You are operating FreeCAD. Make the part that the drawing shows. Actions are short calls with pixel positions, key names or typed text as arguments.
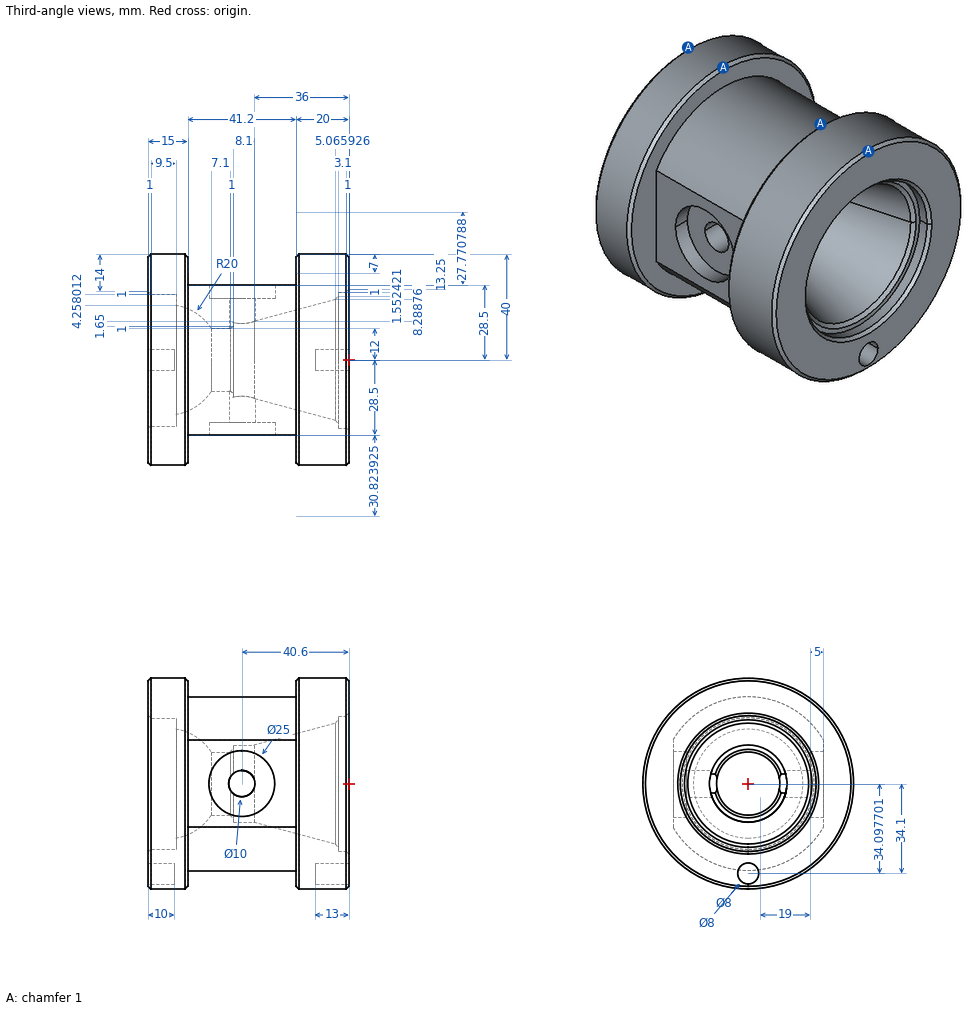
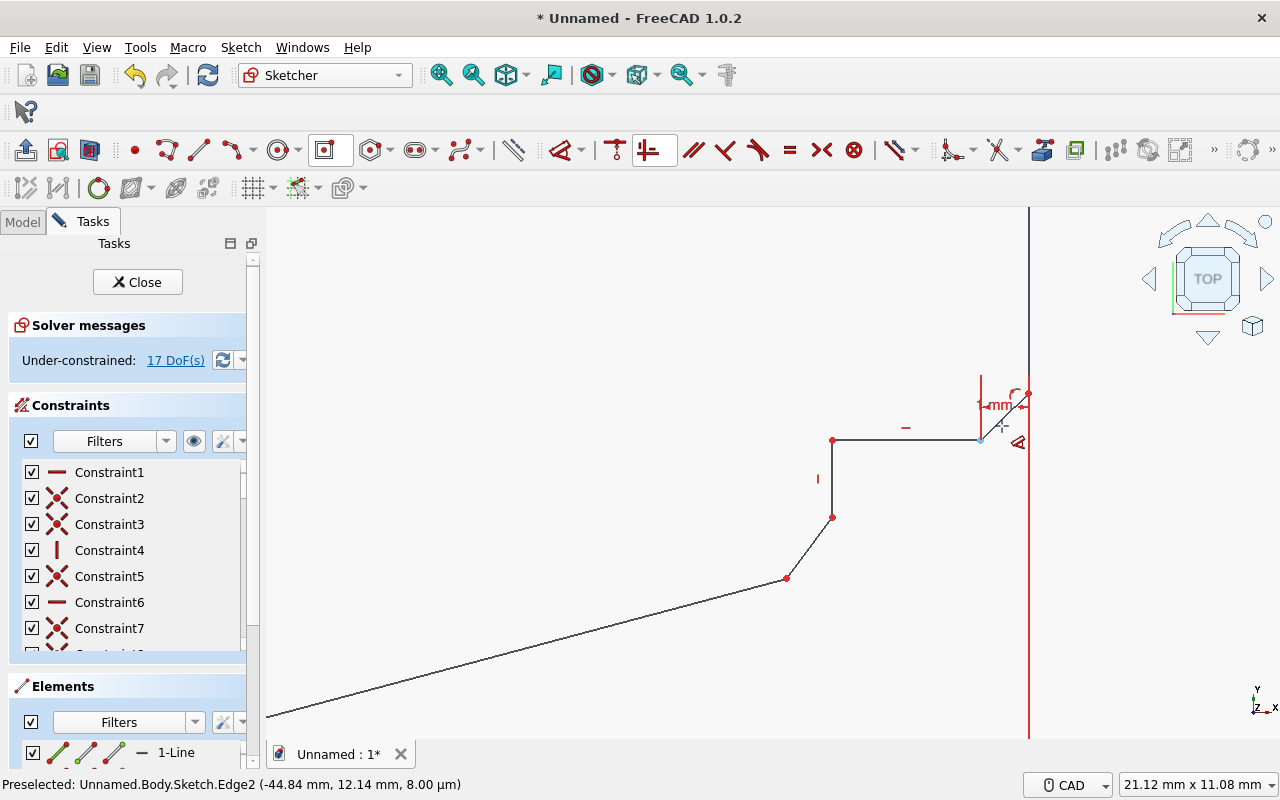
click(995, 426)
click(1063, 428)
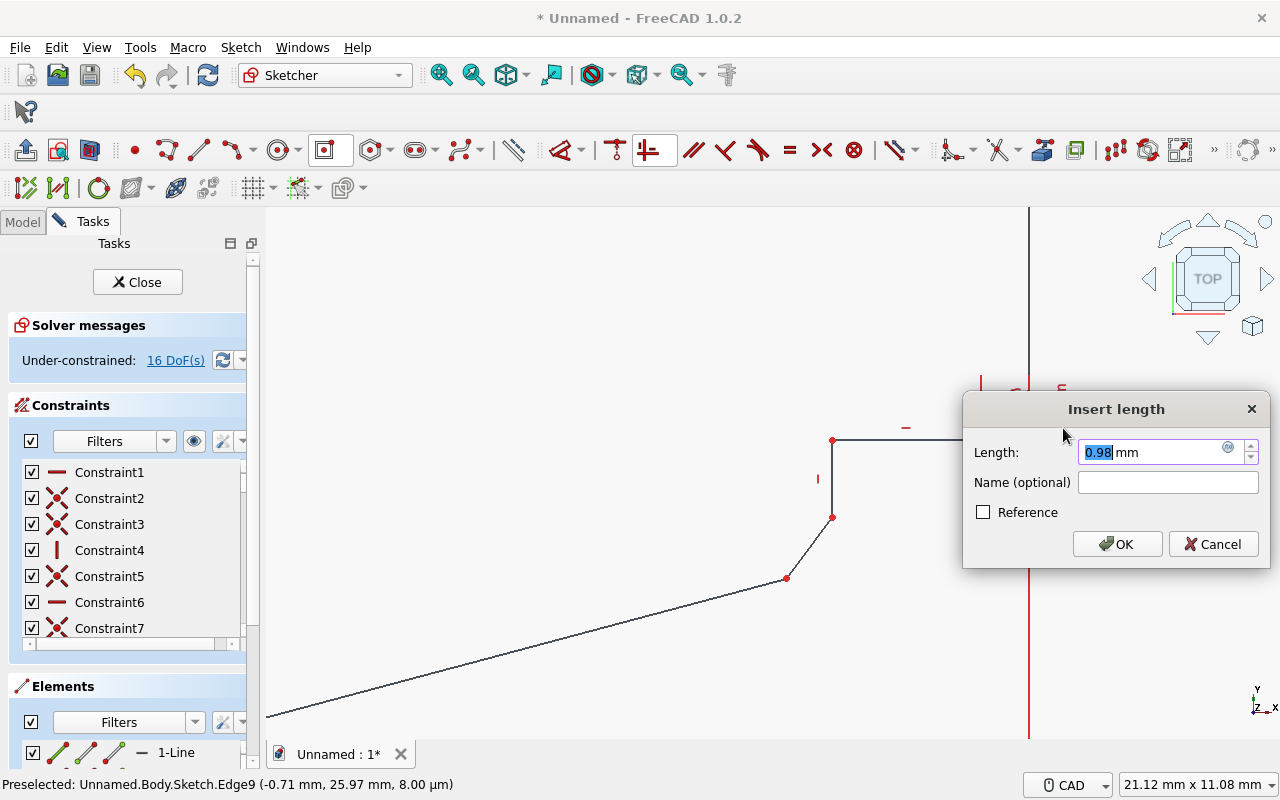
text(1)
key(Return)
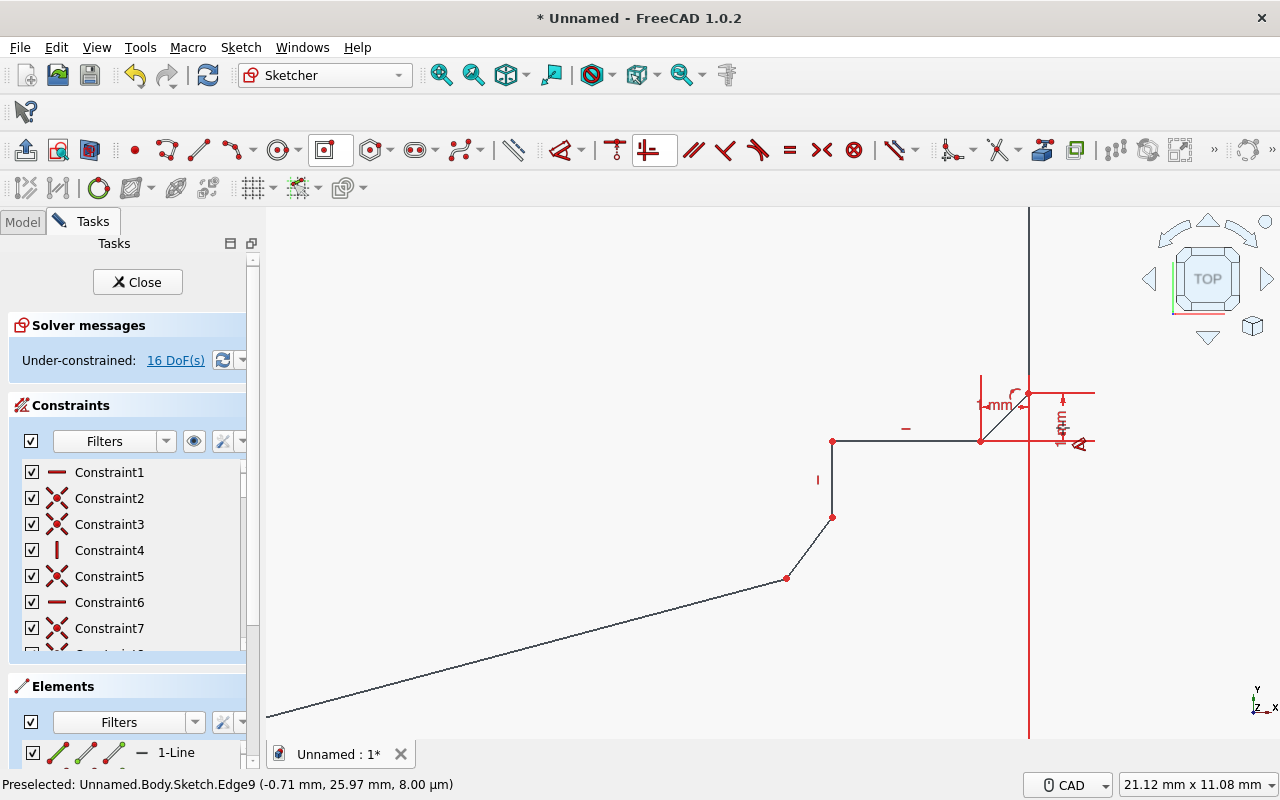
scroll(1003, 425, down, 9)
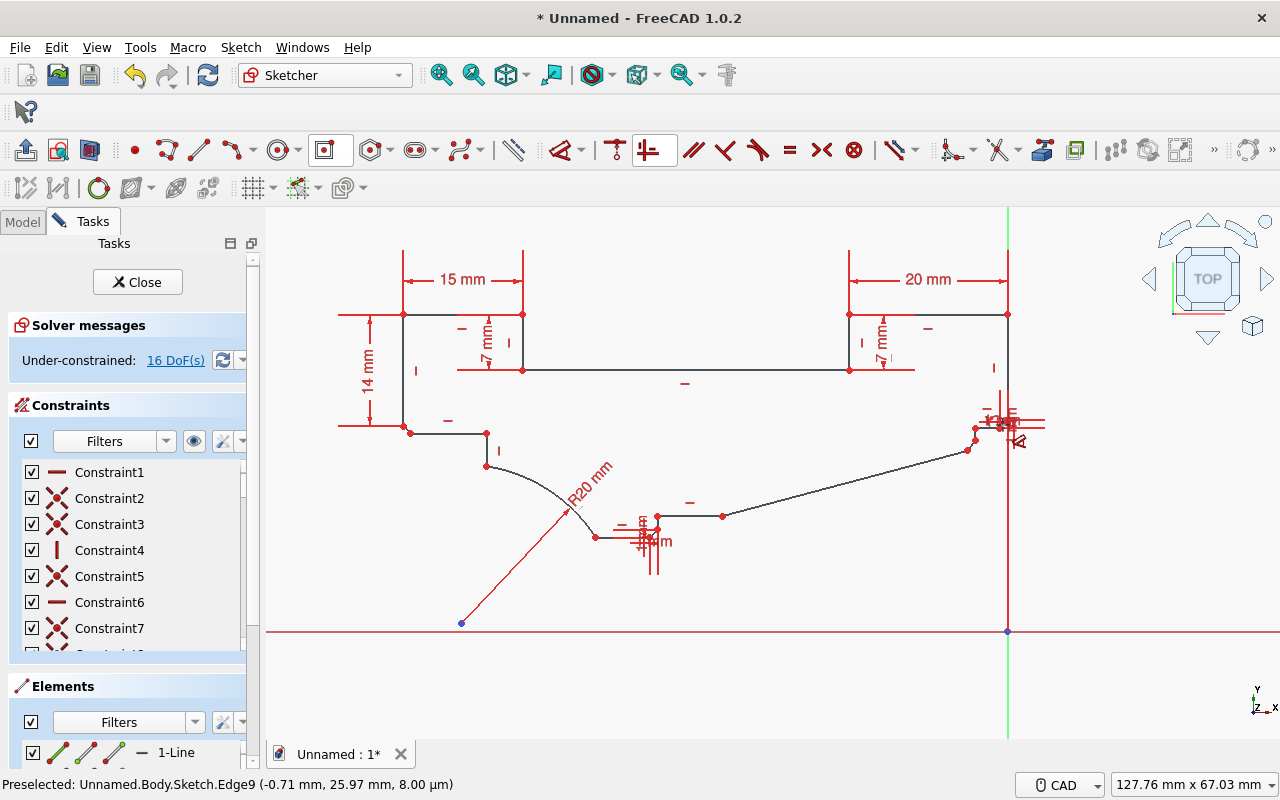
scroll(406, 428, up, 9)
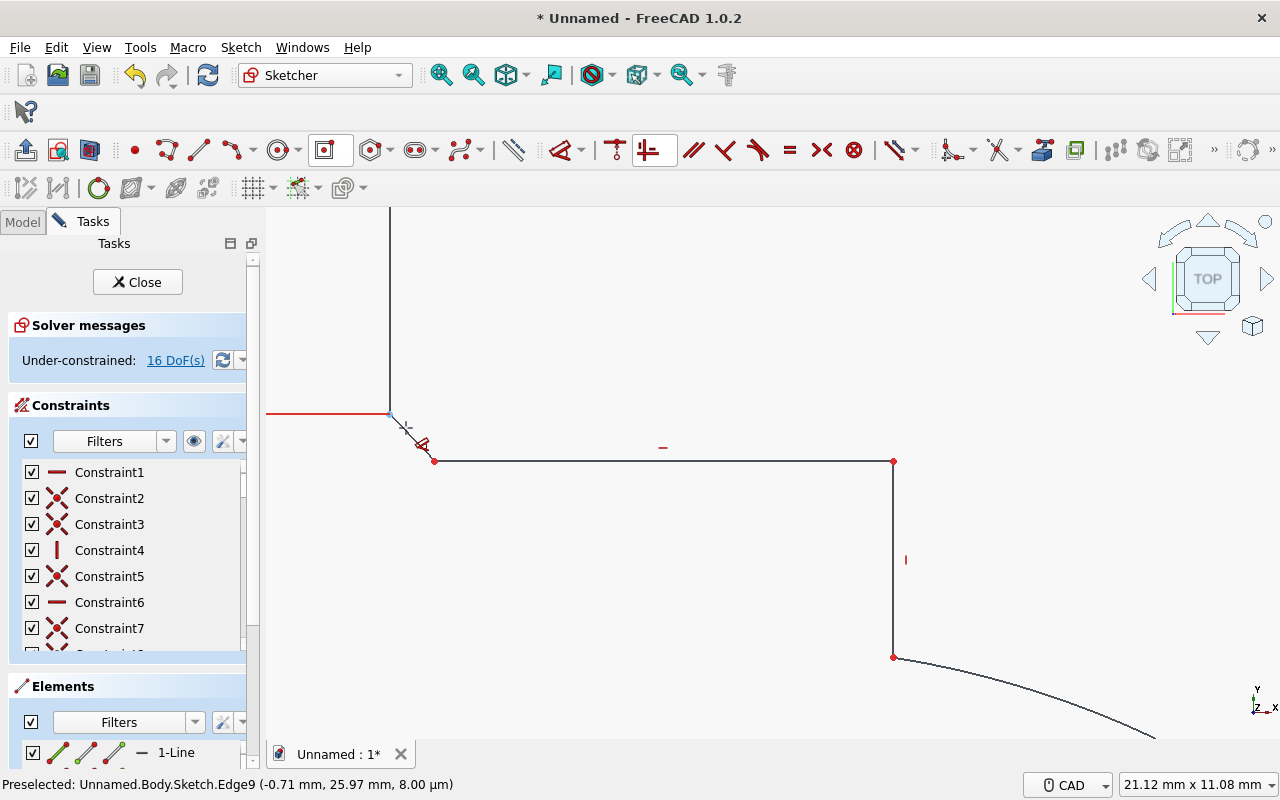
click(403, 428)
click(412, 380)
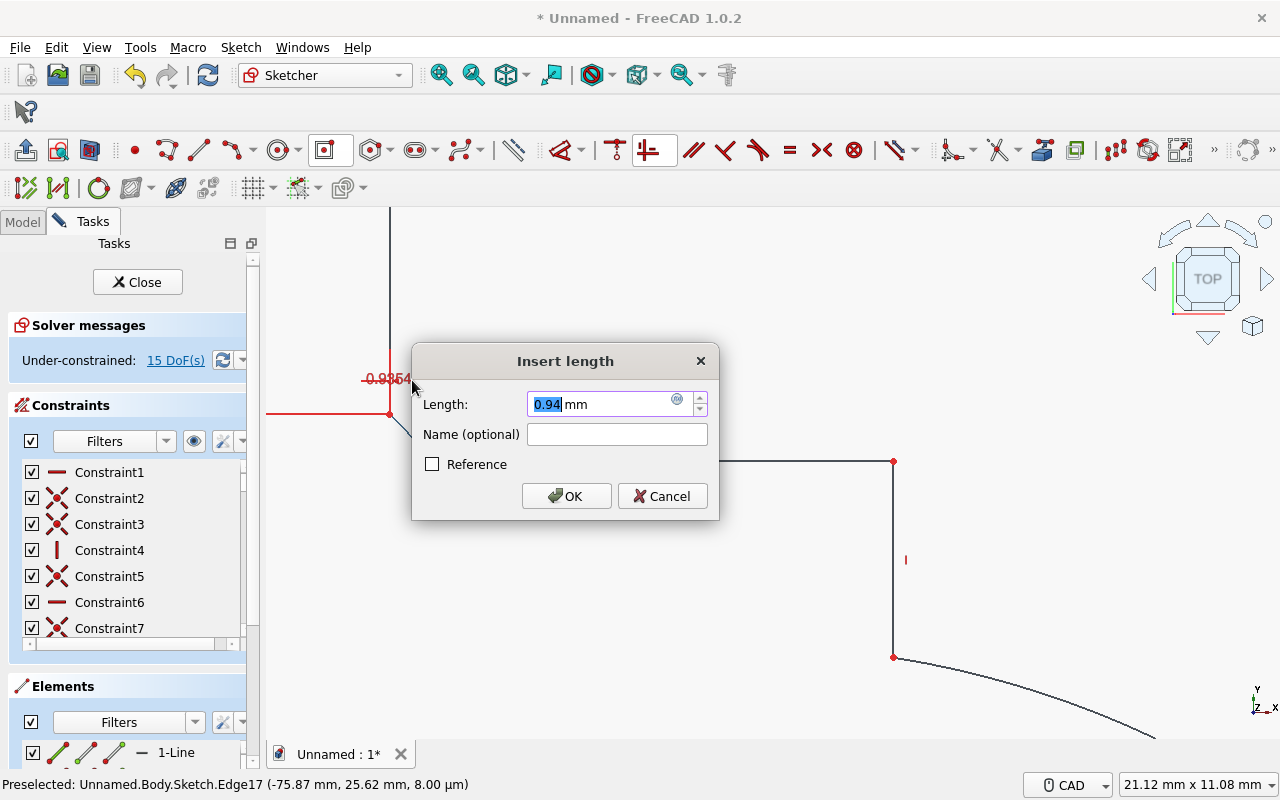
text(1)
key(Return)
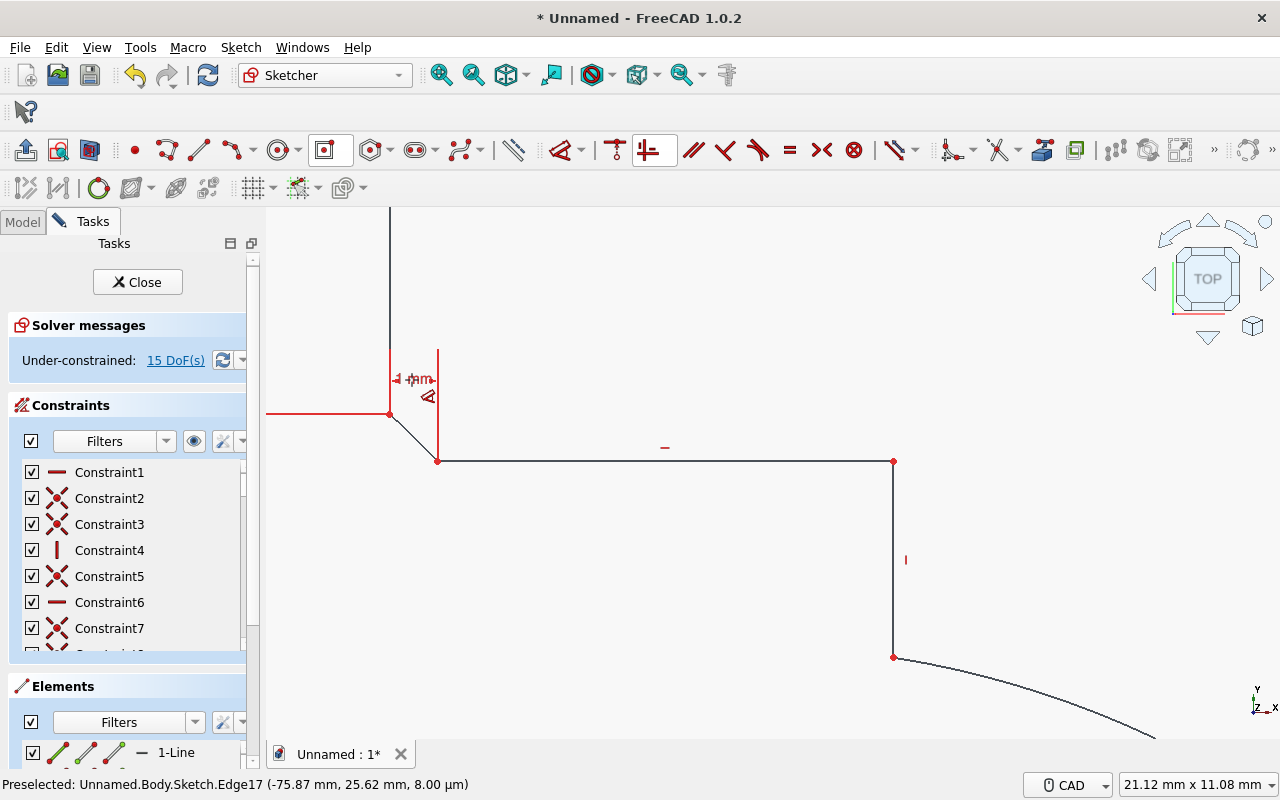
click(404, 428)
click(356, 438)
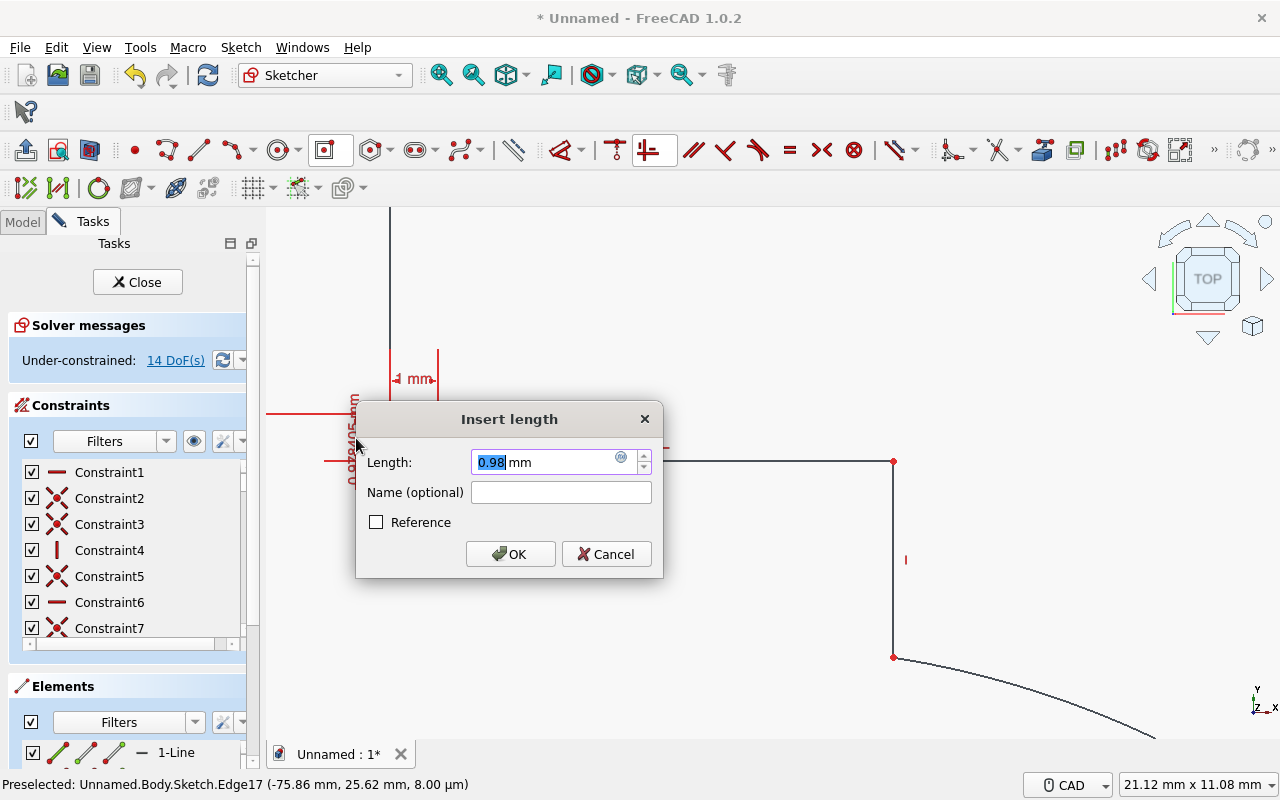
text(1)
key(Return)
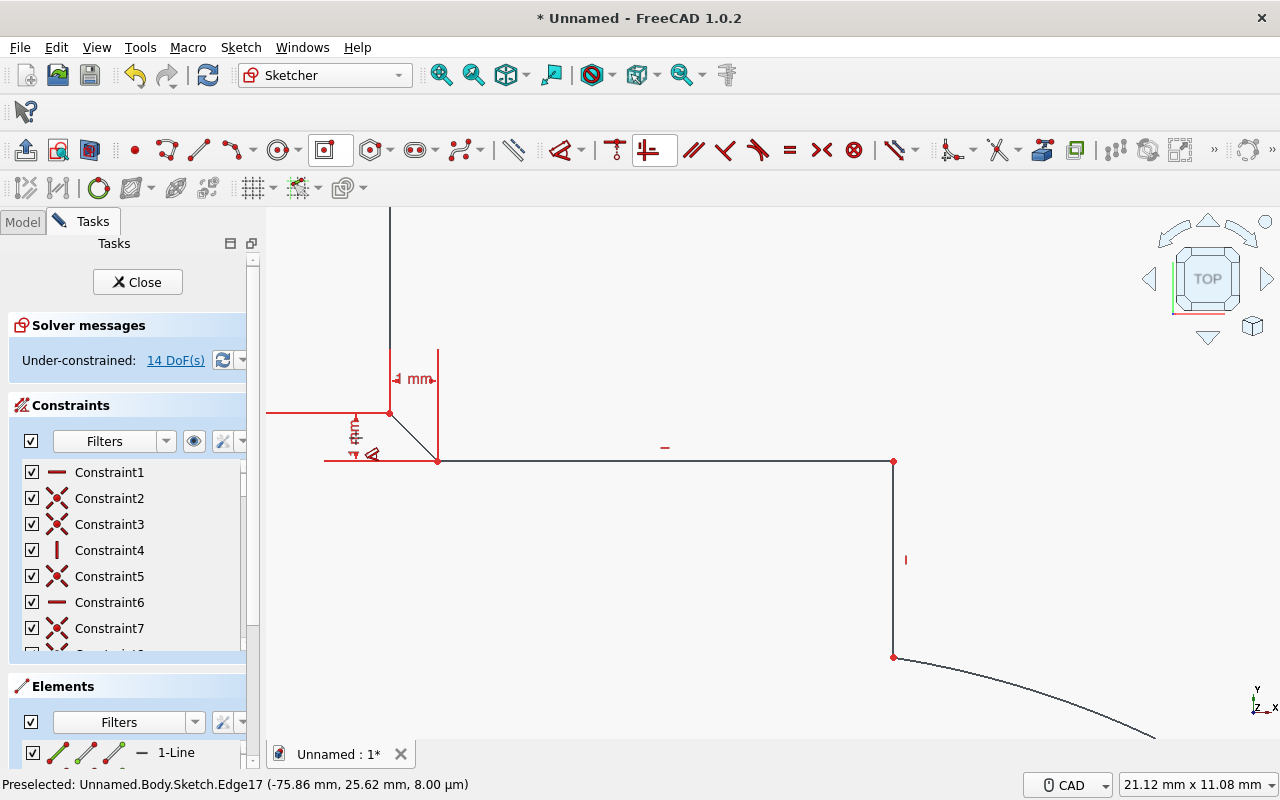
scroll(405, 428, down, 9)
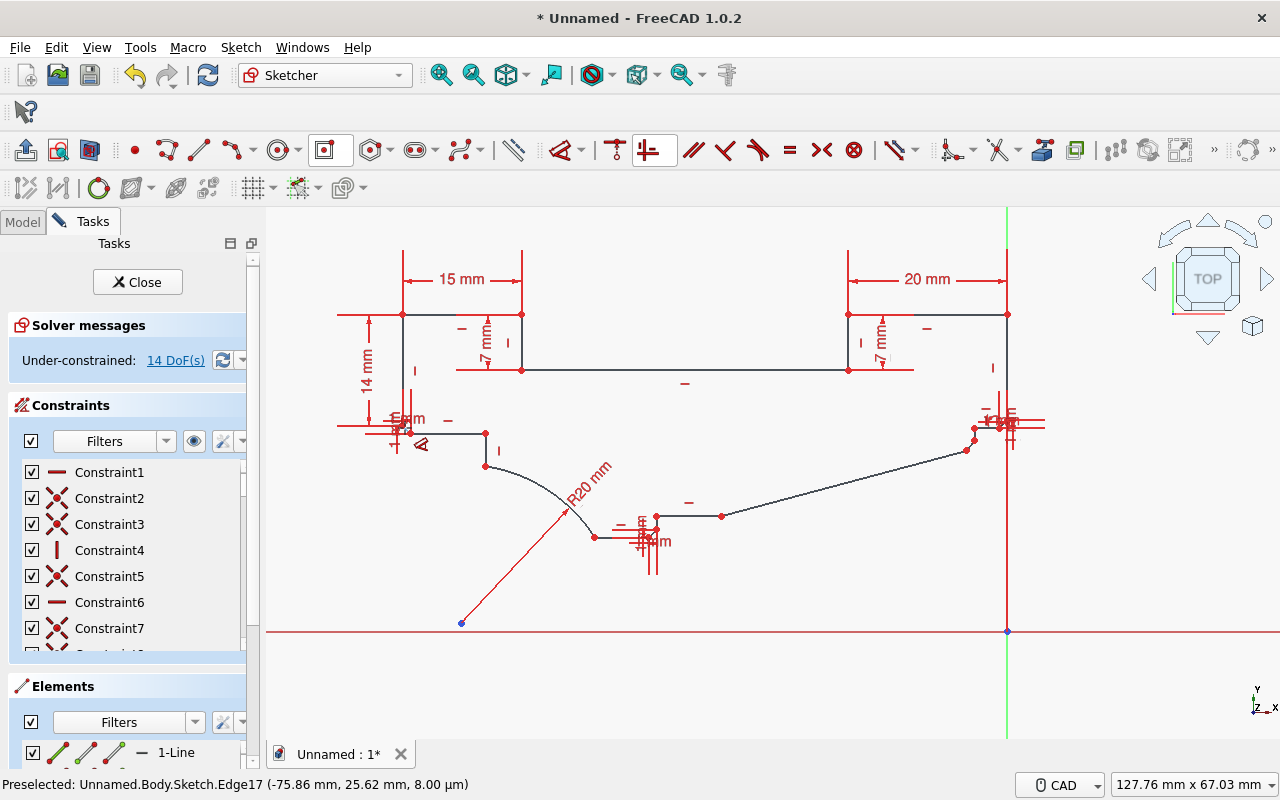
click(611, 538)
click(622, 572)